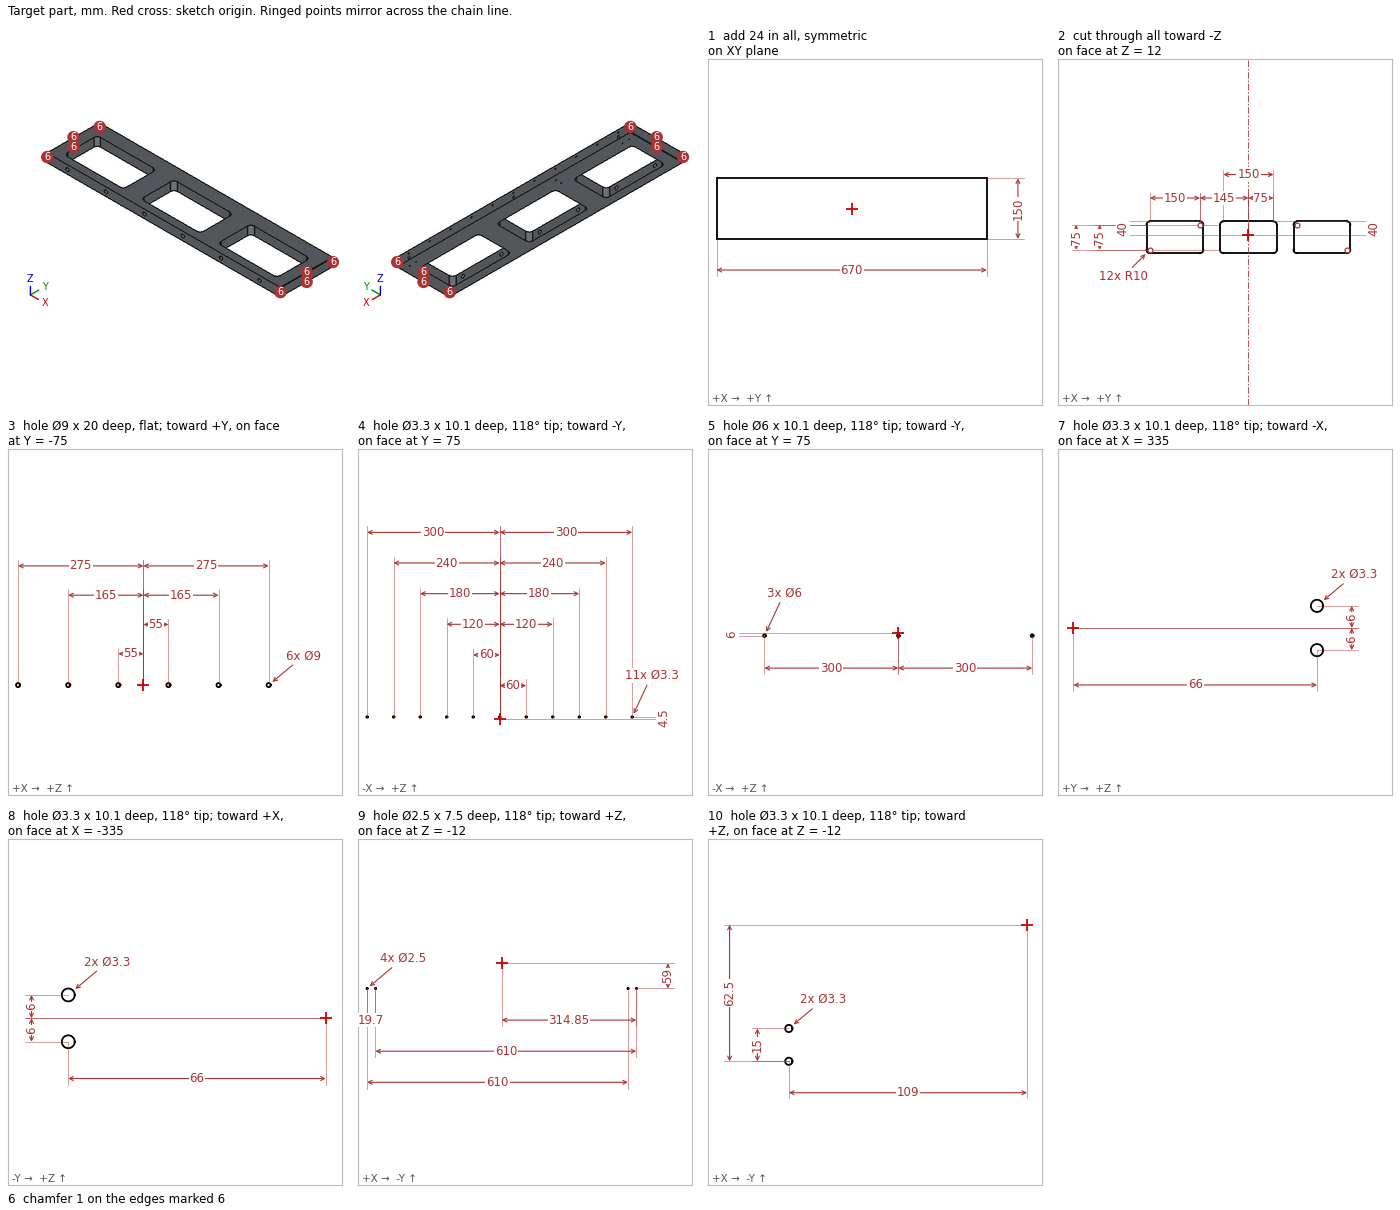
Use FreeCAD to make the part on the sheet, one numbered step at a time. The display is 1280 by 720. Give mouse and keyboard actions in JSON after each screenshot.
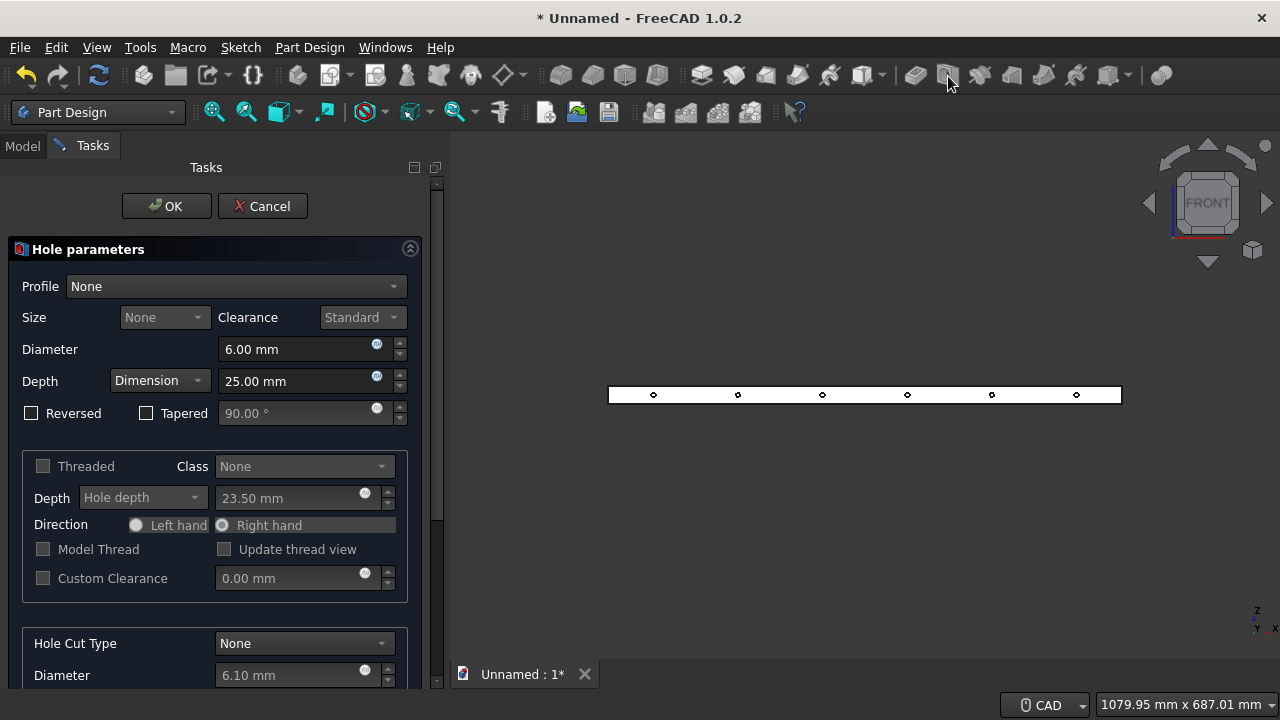
{"action": "triple_click", "coordinate": [305, 349]}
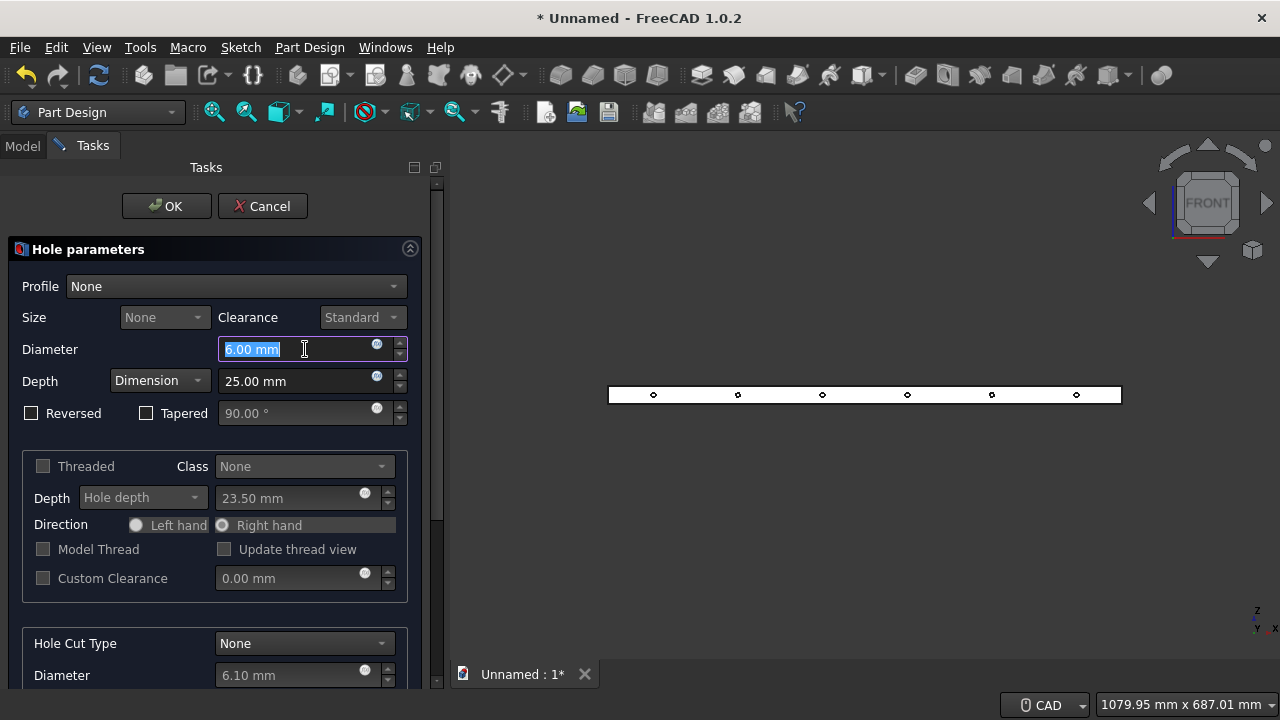
{"action": "type", "text": "9"}
{"action": "key", "text": "Tab"}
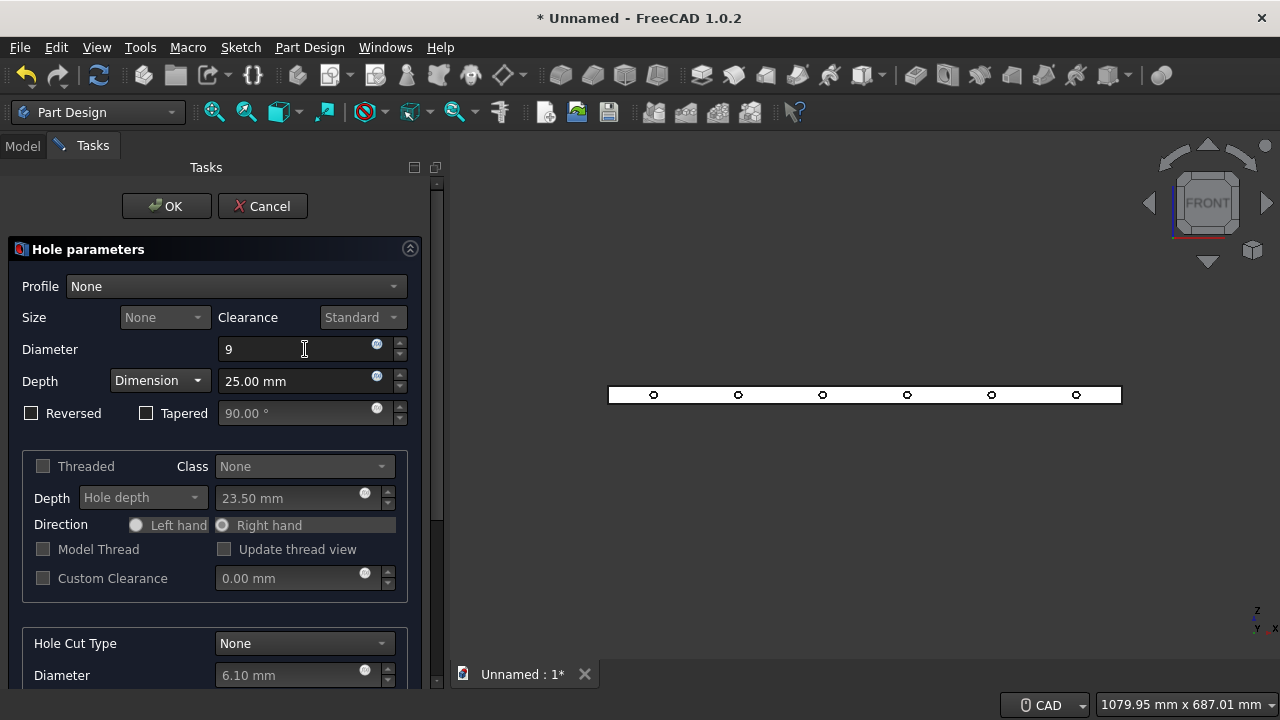
{"action": "triple_click", "coordinate": [305, 381]}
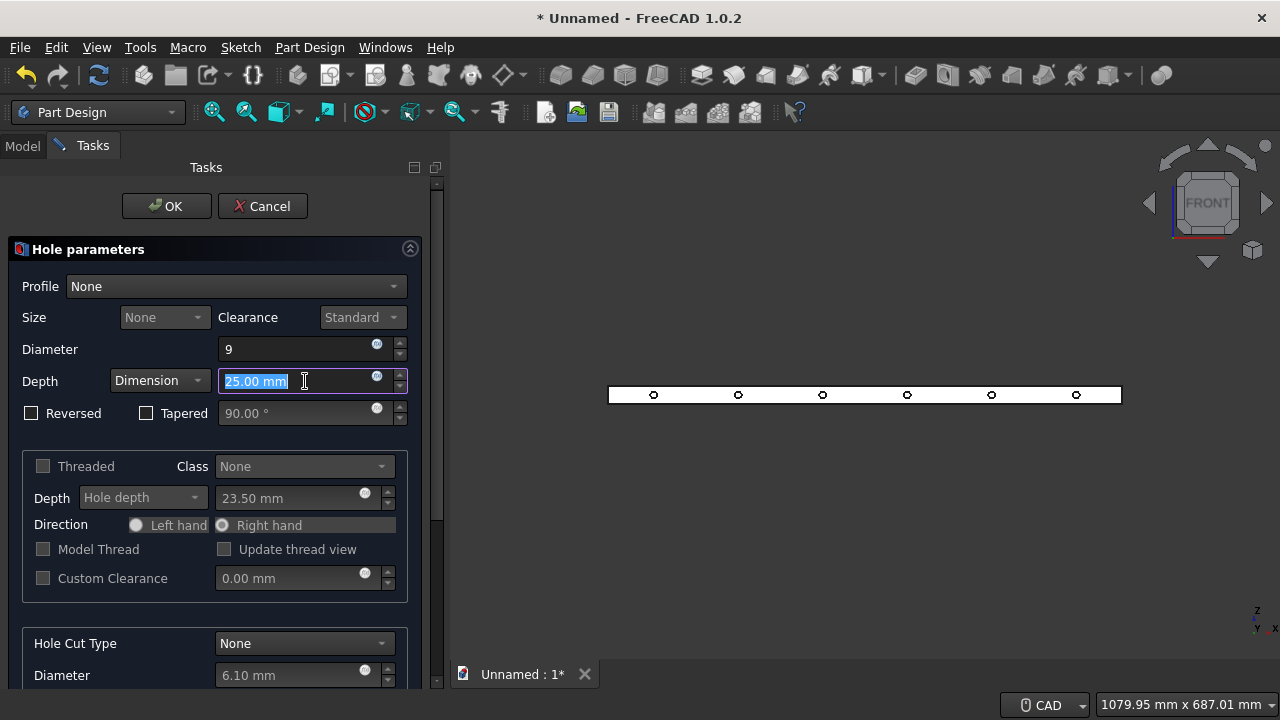
{"action": "type", "text": "20"}
{"action": "key", "text": "Tab"}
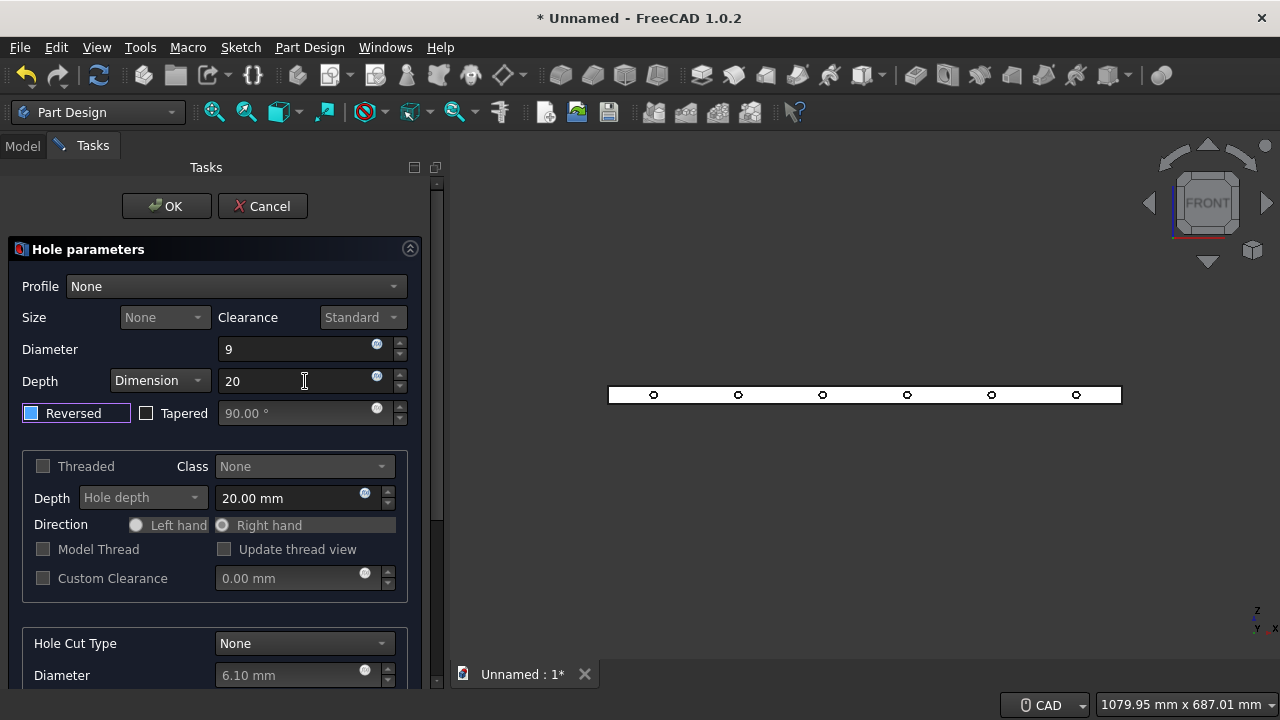
{"action": "scroll", "coordinate": [437, 432], "scroll_direction": "down", "scroll_amount": 4}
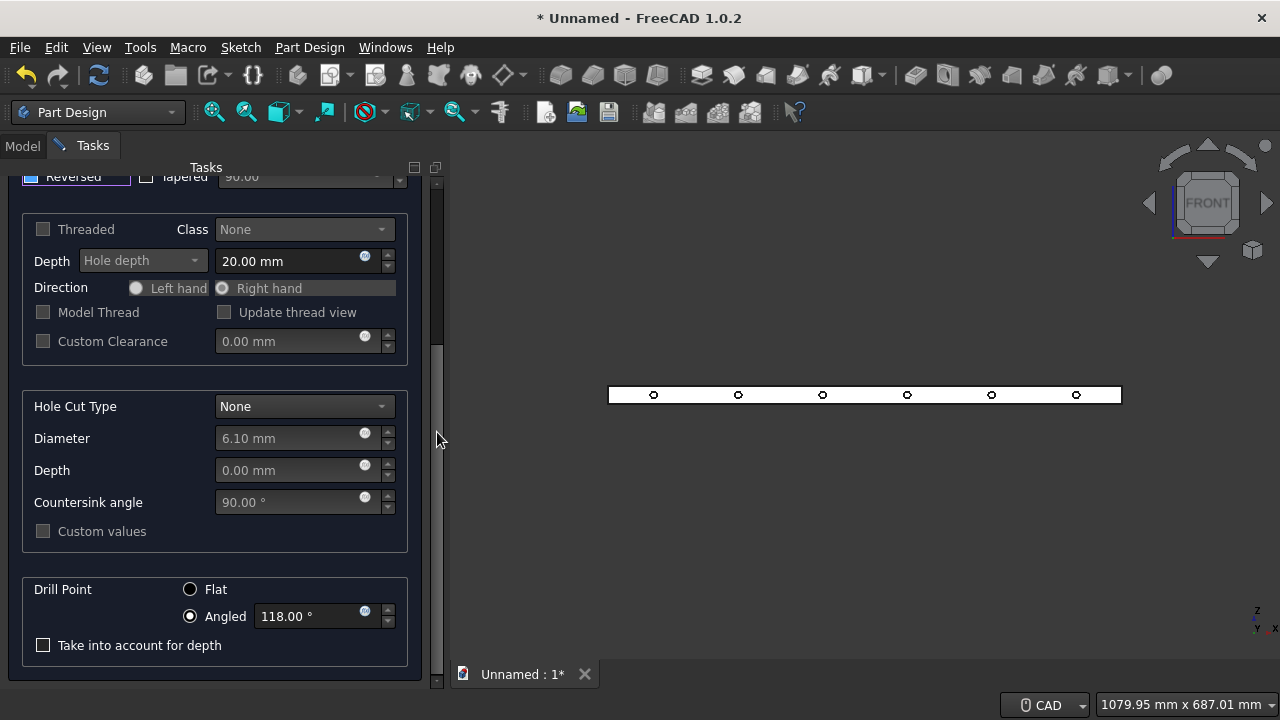
{"action": "left_click", "coordinate": [191, 589]}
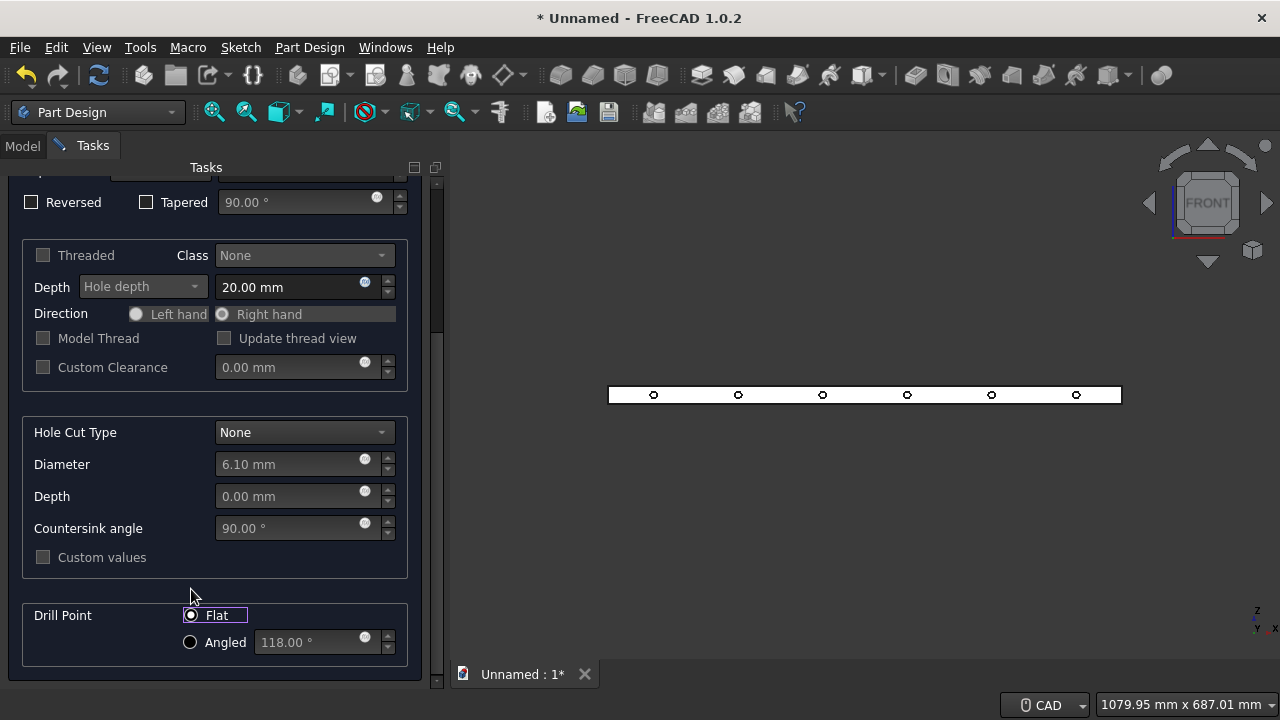
{"action": "scroll", "coordinate": [437, 432], "scroll_direction": "up", "scroll_amount": 5}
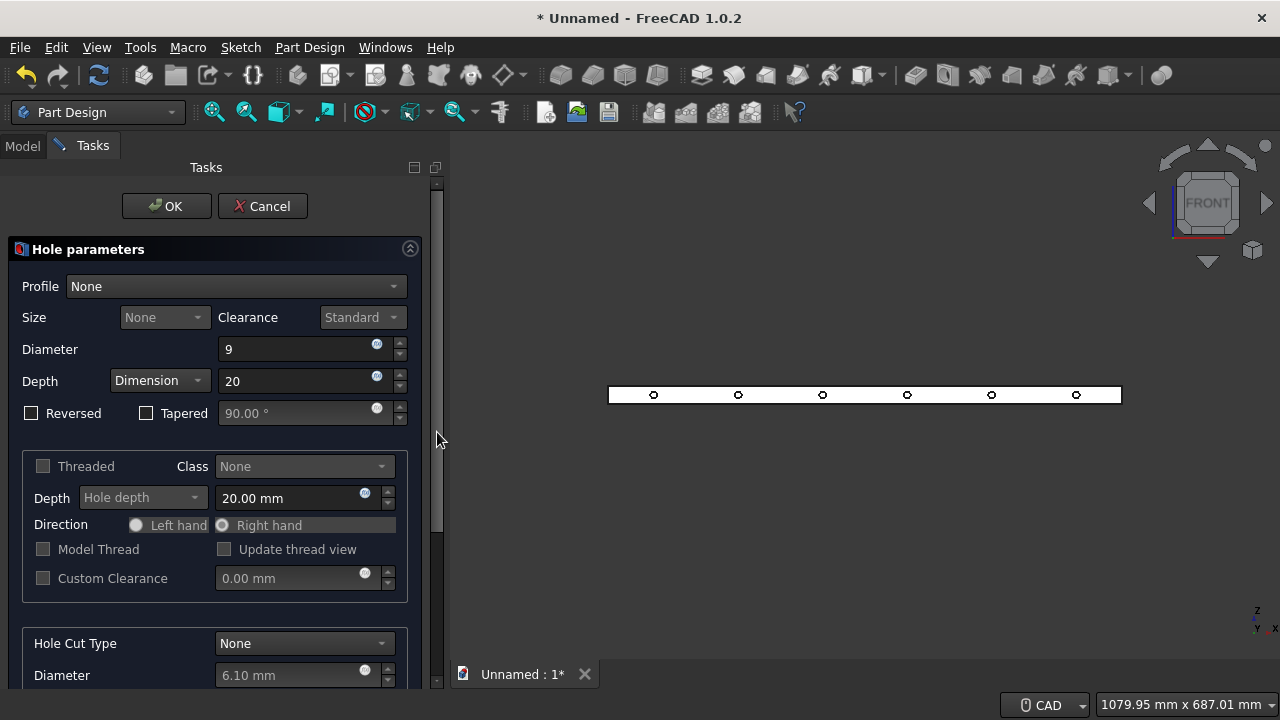
{"action": "left_click", "coordinate": [167, 206]}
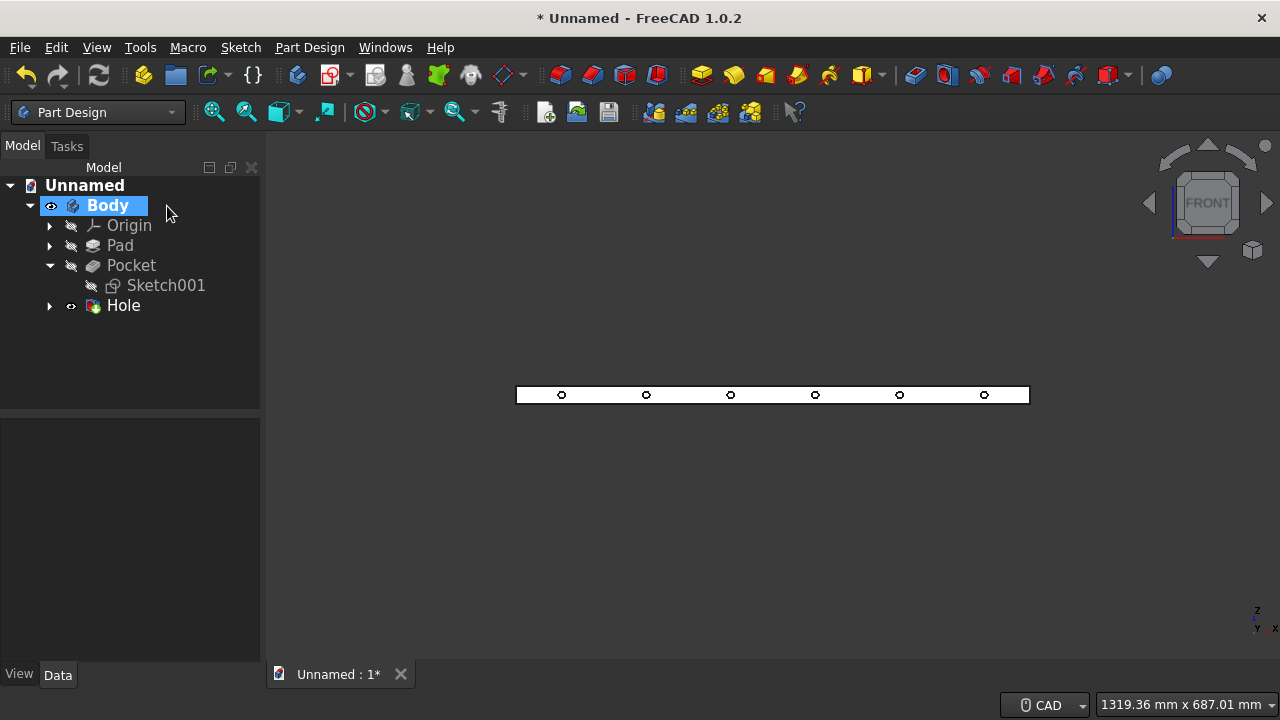
{"action": "key", "text": "4"}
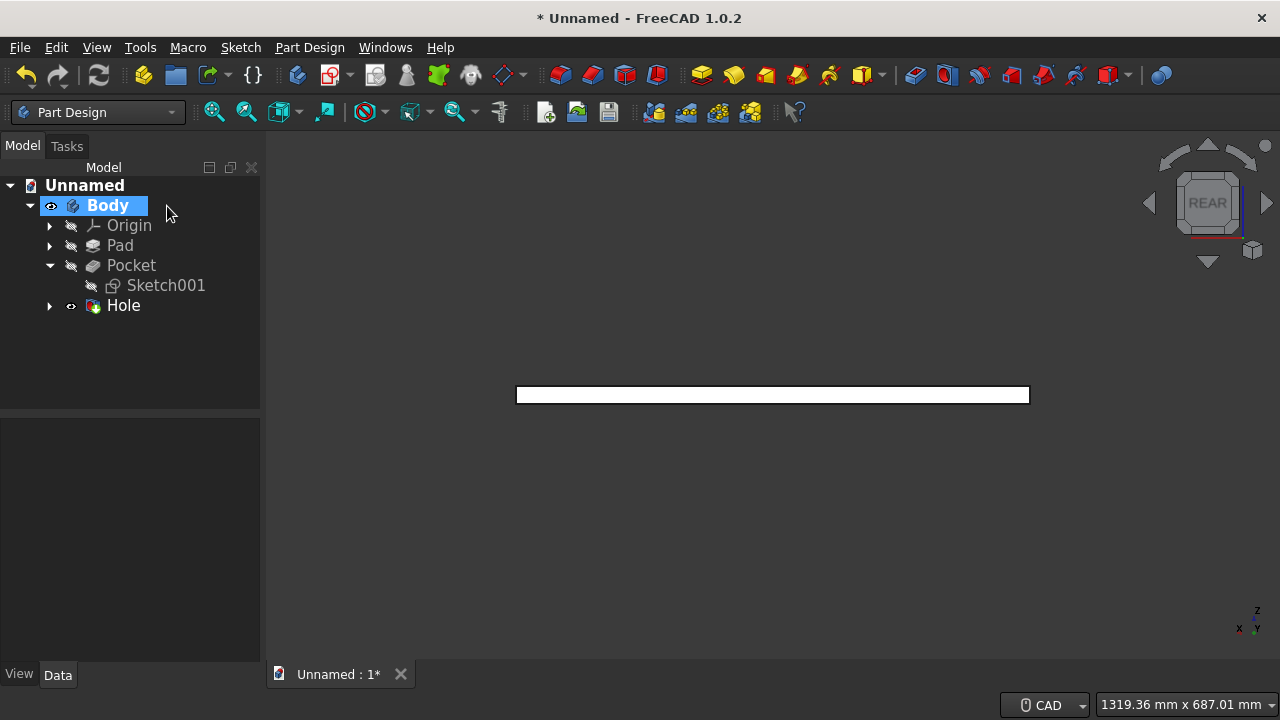
{"action": "left_click", "coordinate": [552, 394]}